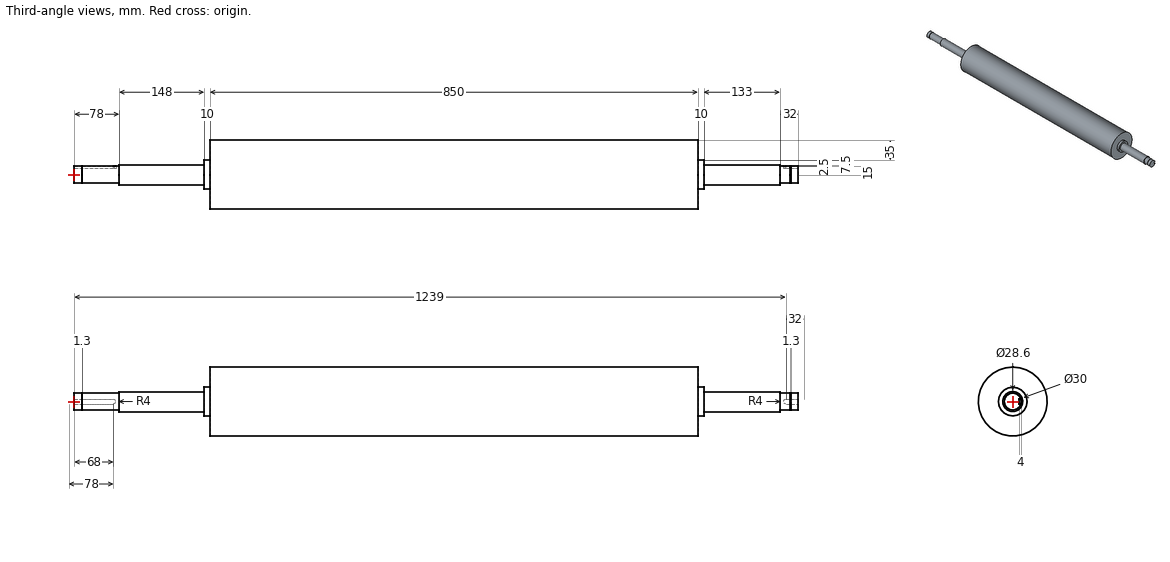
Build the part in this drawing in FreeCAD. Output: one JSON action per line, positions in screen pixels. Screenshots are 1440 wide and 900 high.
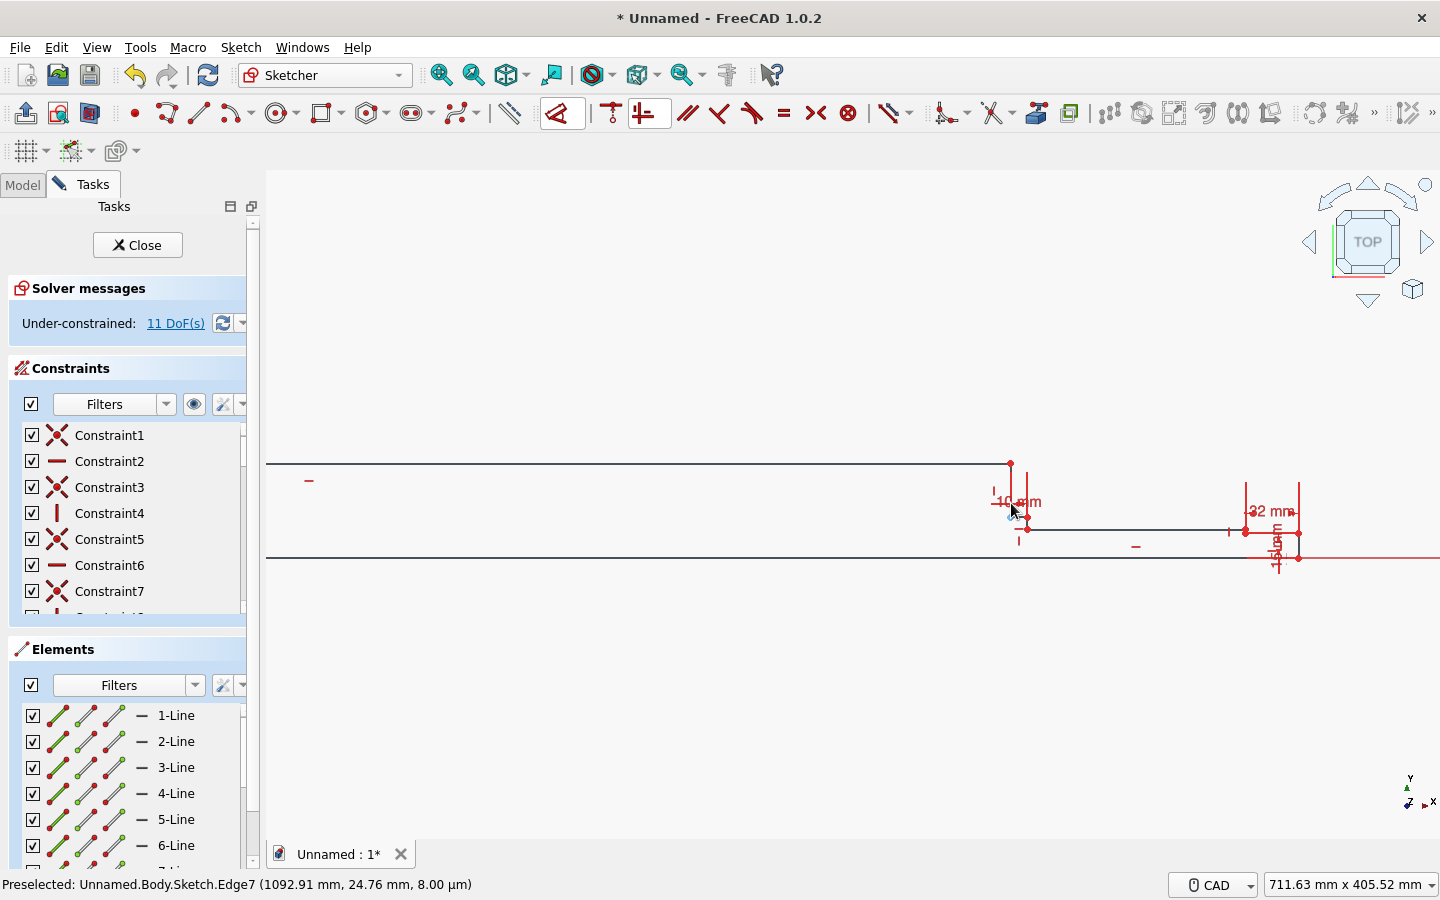
{"action": "left_click", "coordinate": [1011, 480]}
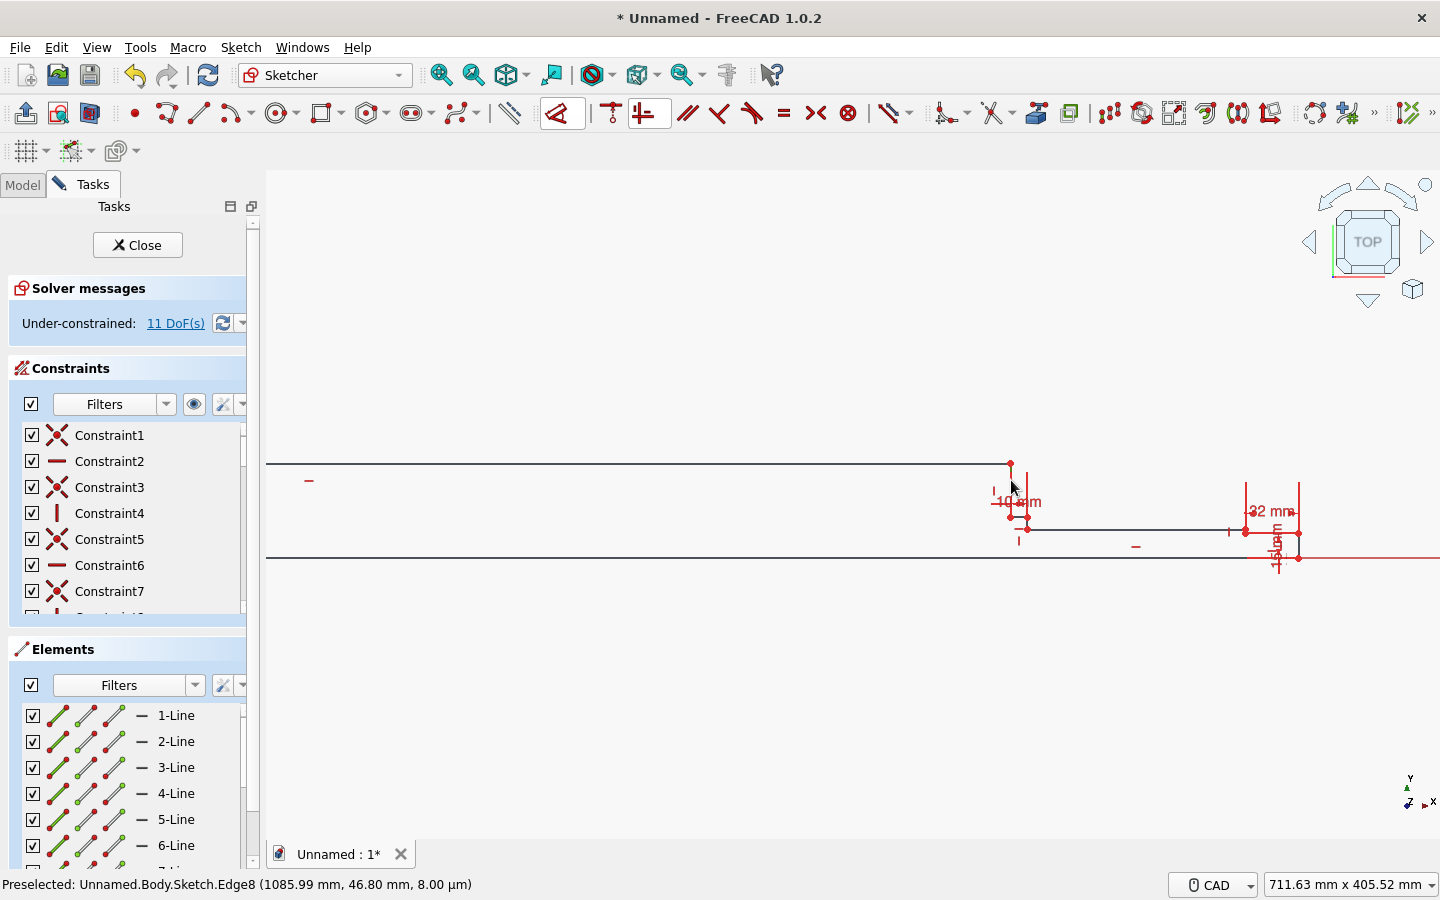
{"action": "key", "text": "i"}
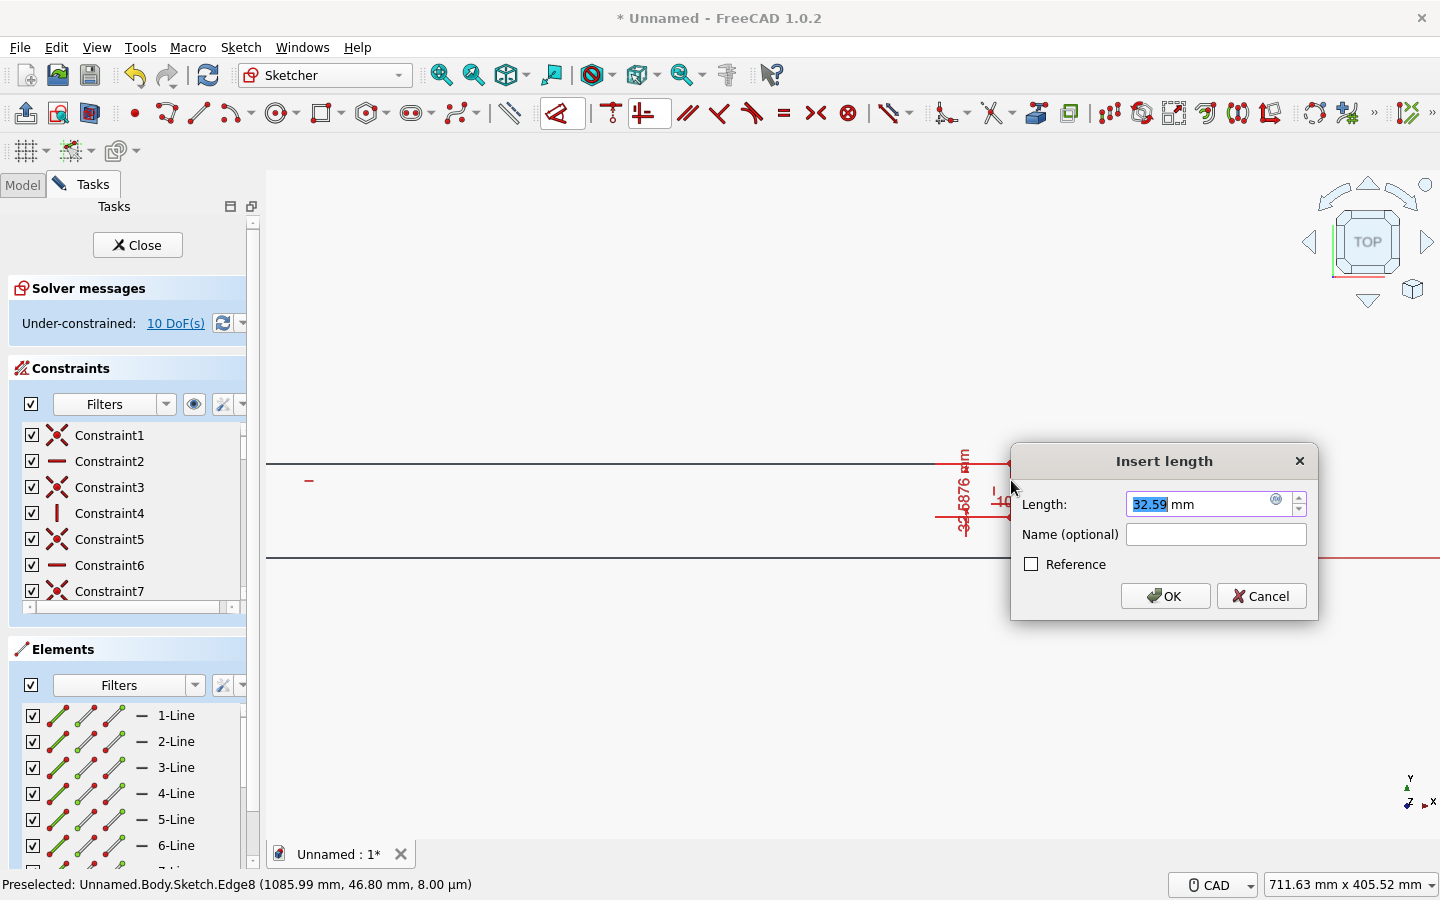
{"action": "type", "text": "35"}
{"action": "key", "text": "Return"}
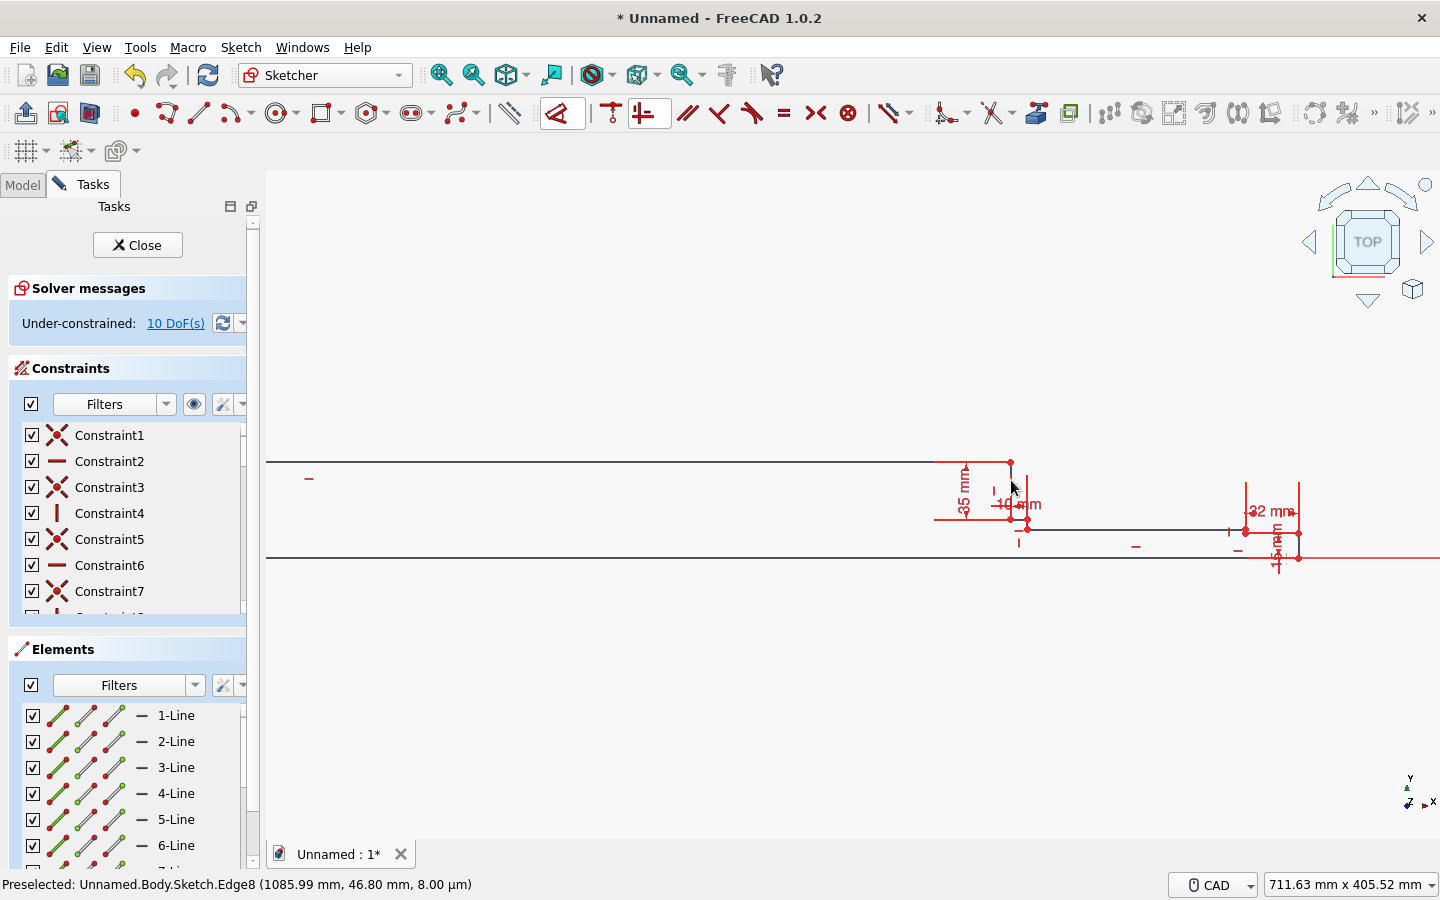
{"action": "scroll", "coordinate": [1011, 503], "scroll_direction": "down", "scroll_amount": 6}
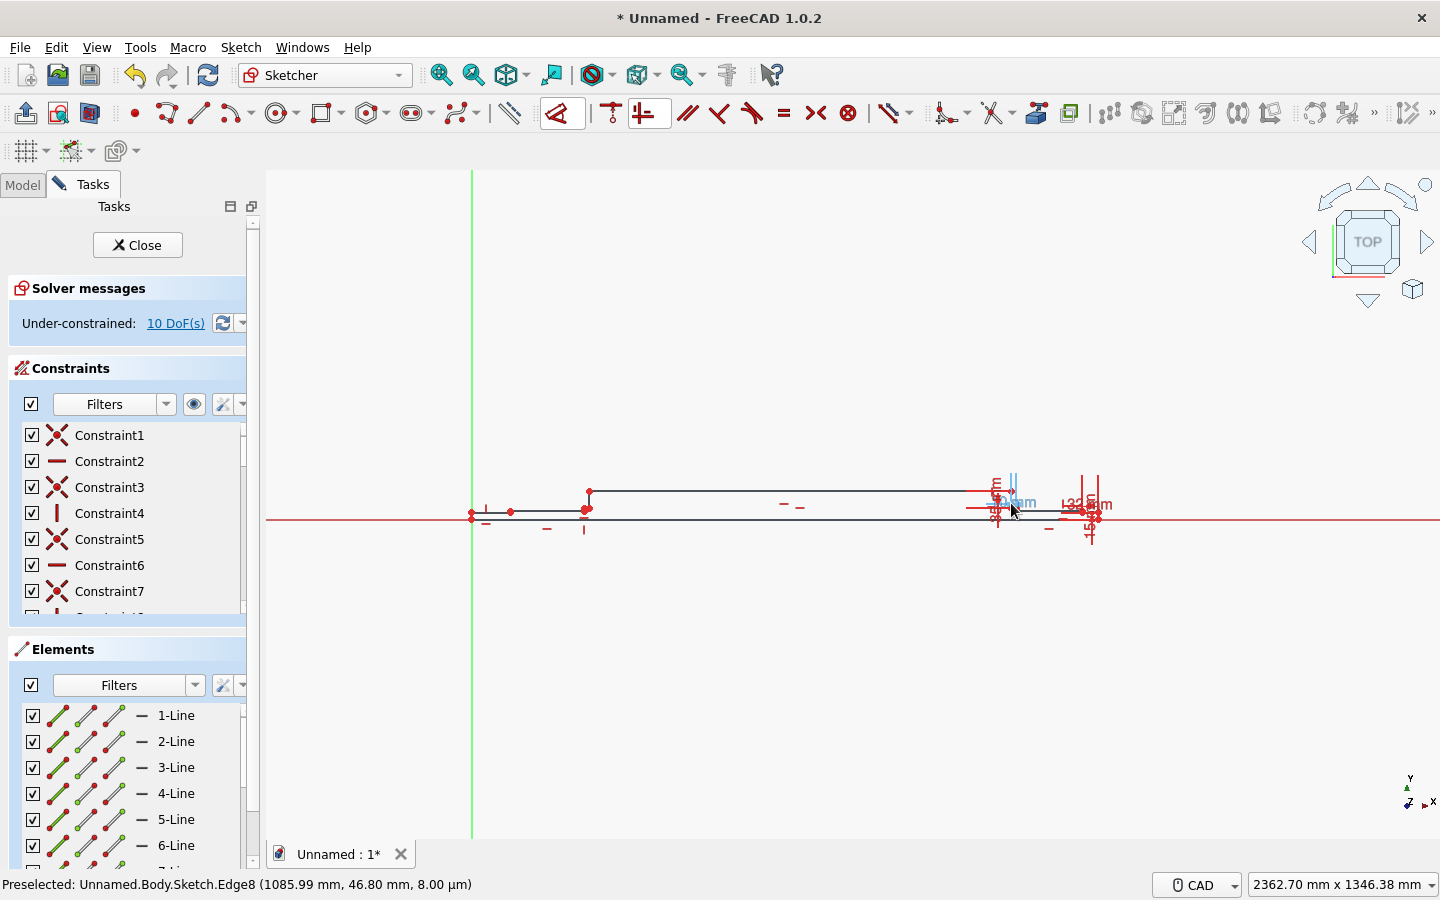
{"action": "scroll", "coordinate": [589, 496], "scroll_direction": "up", "scroll_amount": 5}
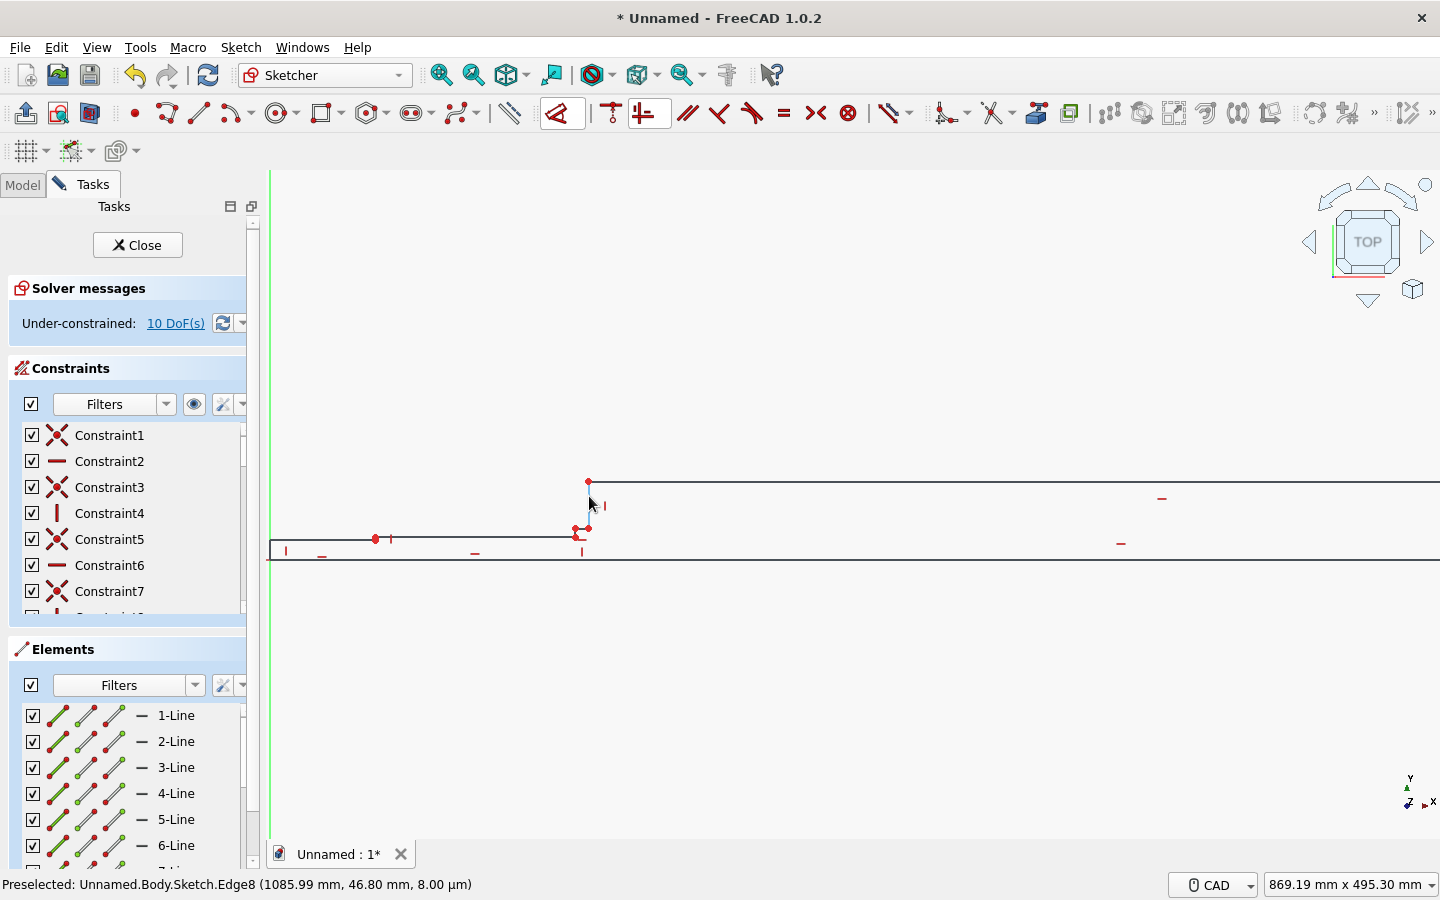
{"action": "left_click", "coordinate": [589, 496]}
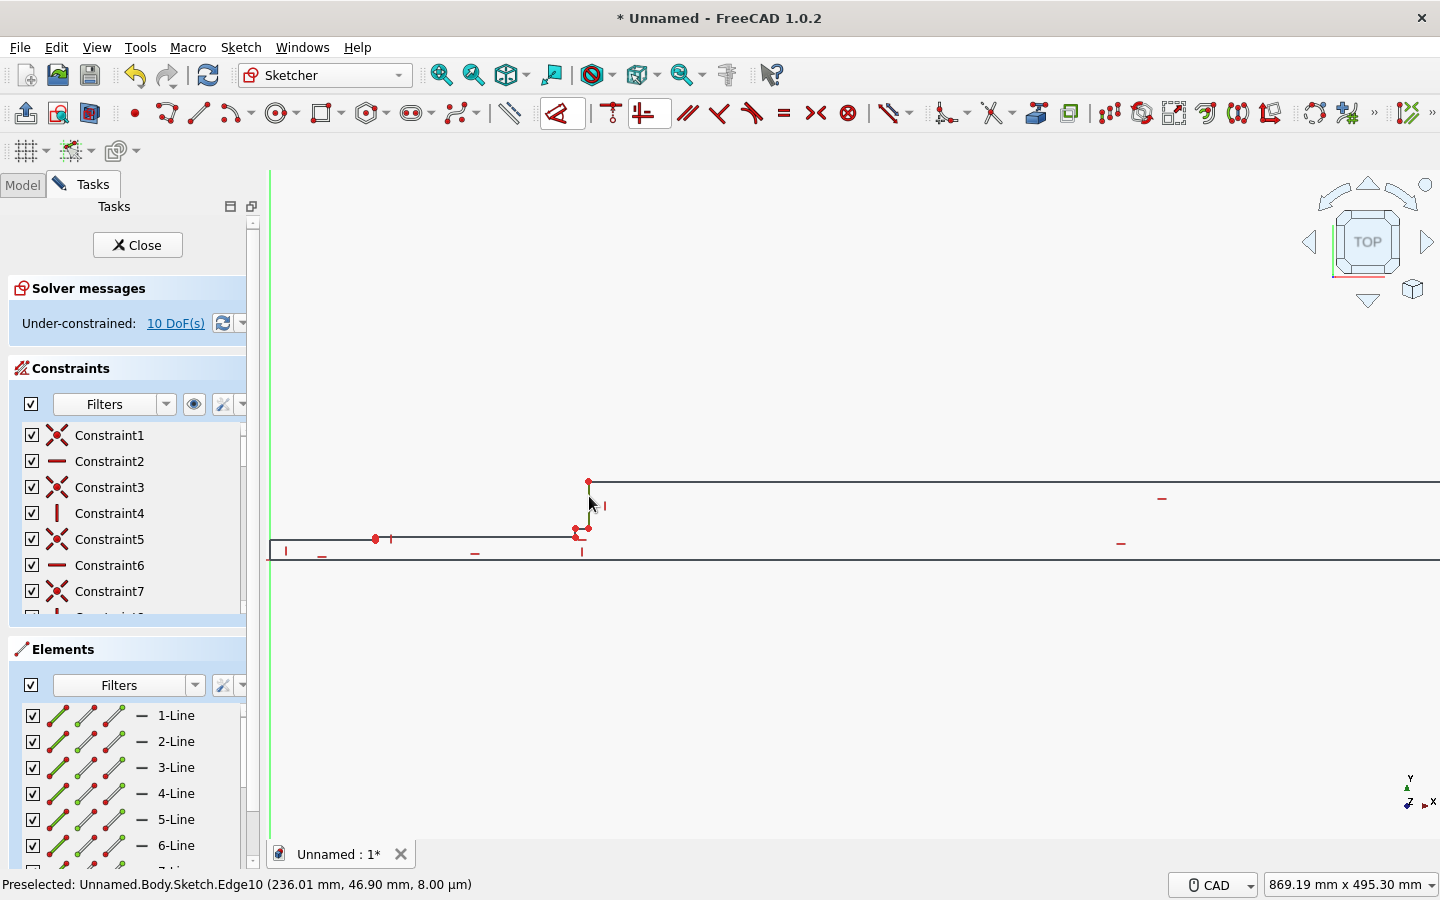
{"action": "left_click", "coordinate": [580, 114]}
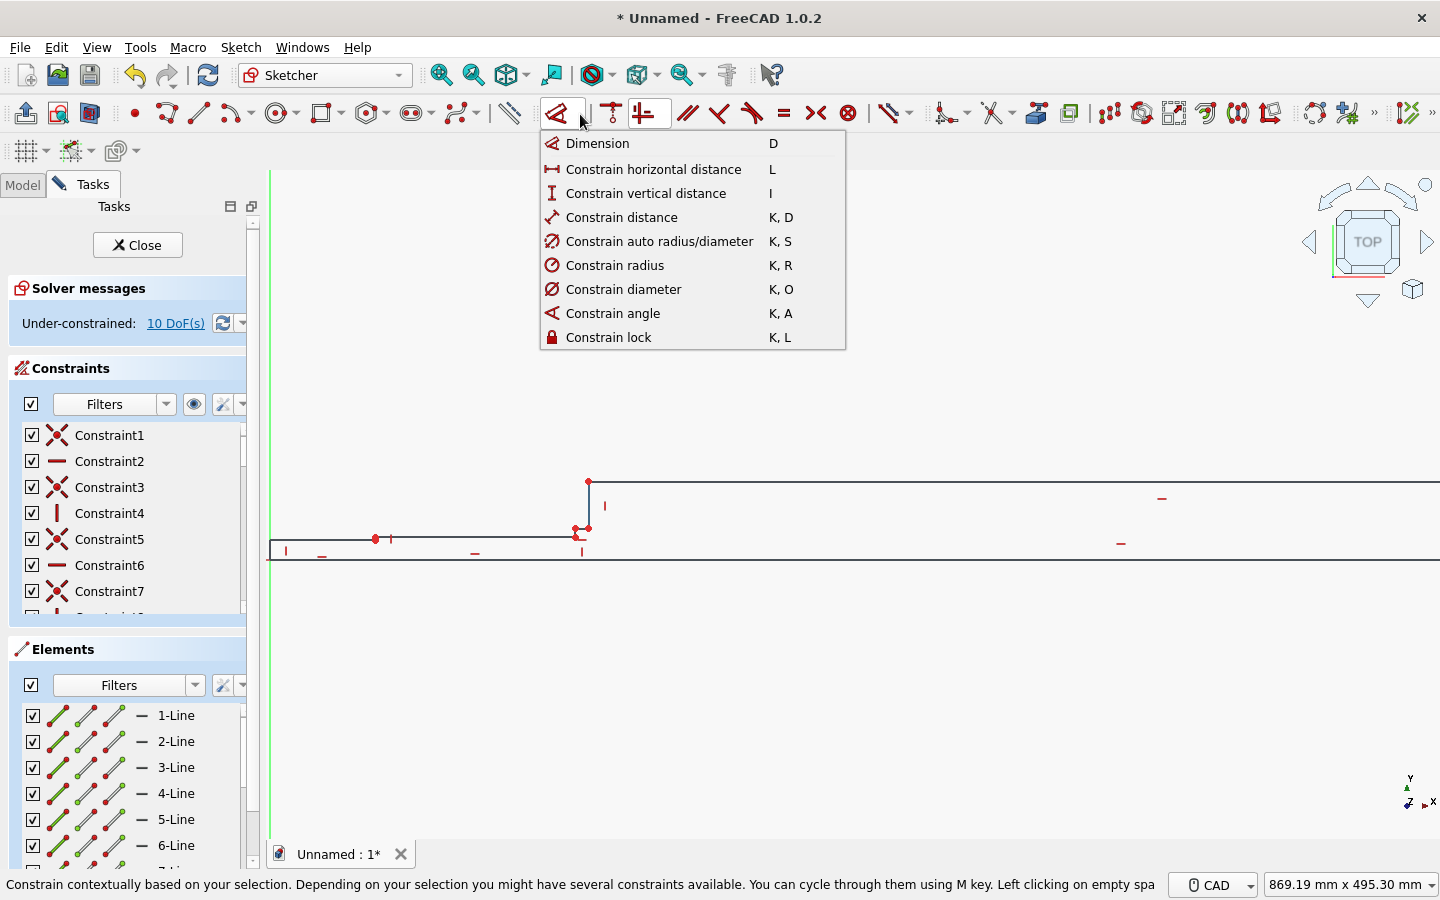
{"action": "left_click", "coordinate": [693, 193]}